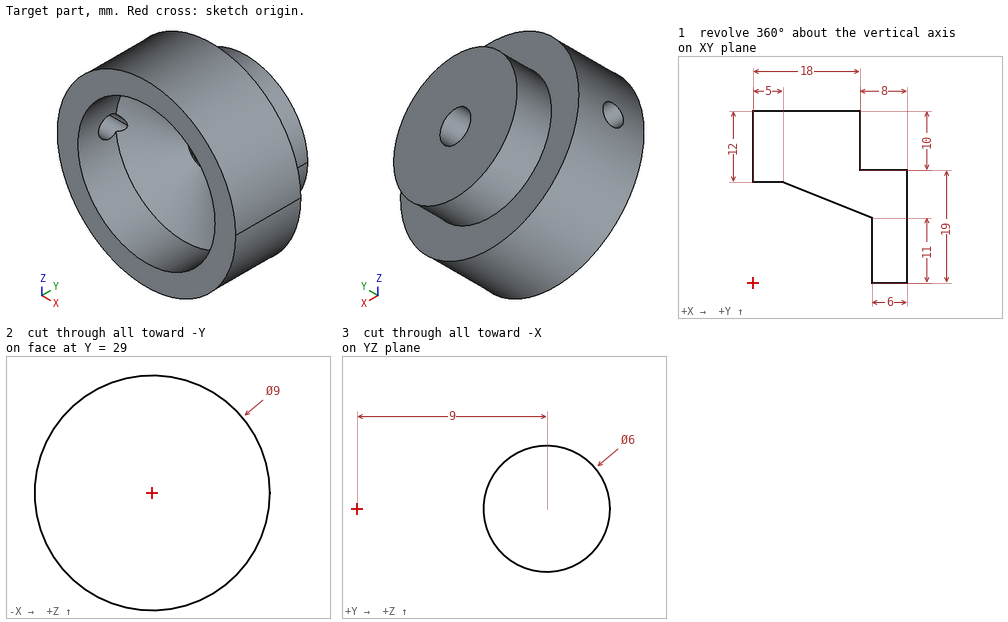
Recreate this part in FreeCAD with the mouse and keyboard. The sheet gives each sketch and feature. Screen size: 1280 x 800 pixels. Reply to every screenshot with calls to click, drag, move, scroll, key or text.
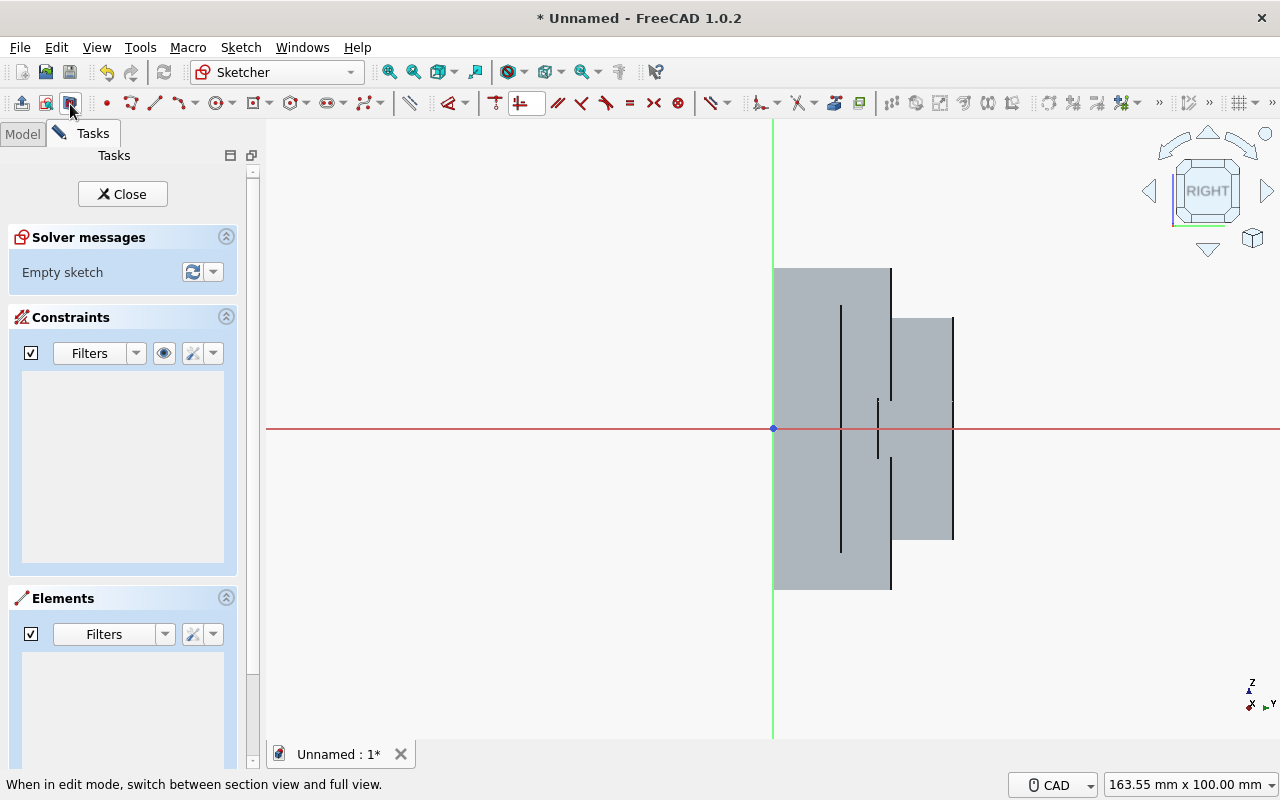
scroll(827, 429, up, 10)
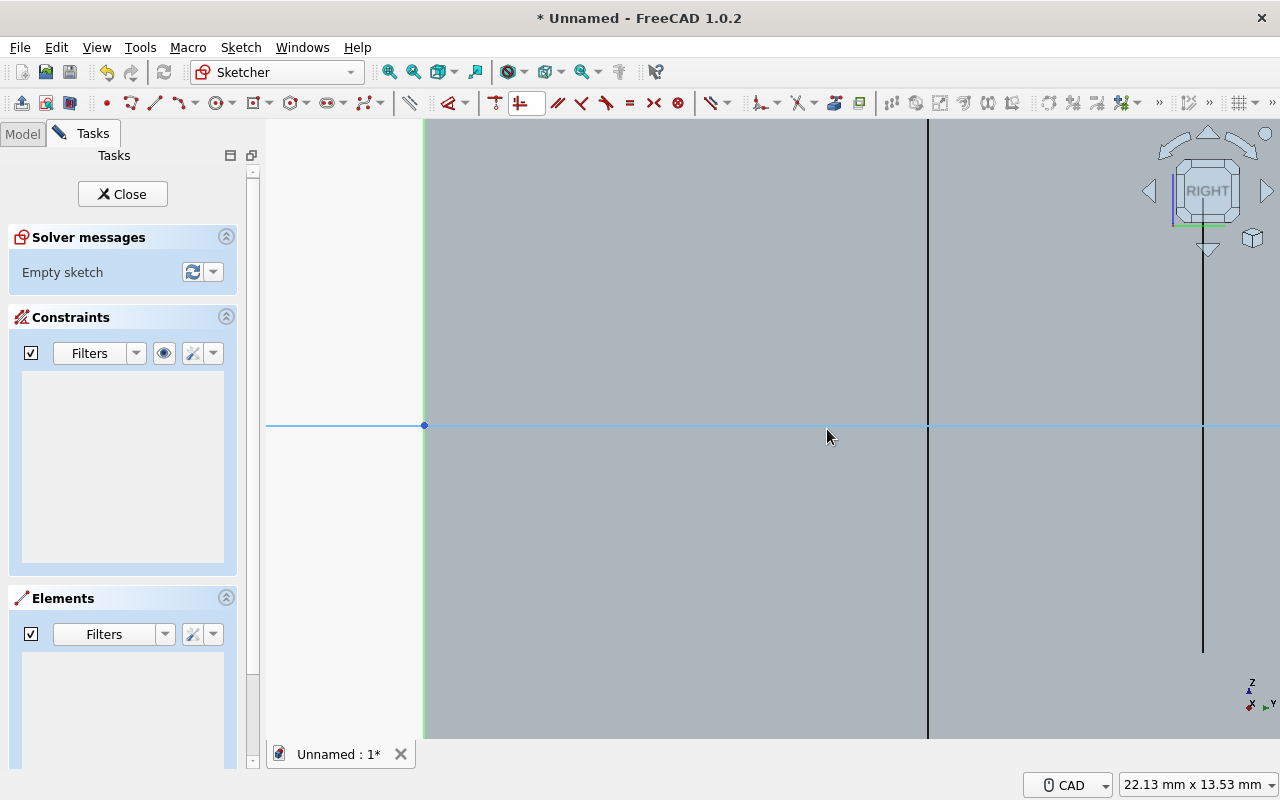
click(216, 104)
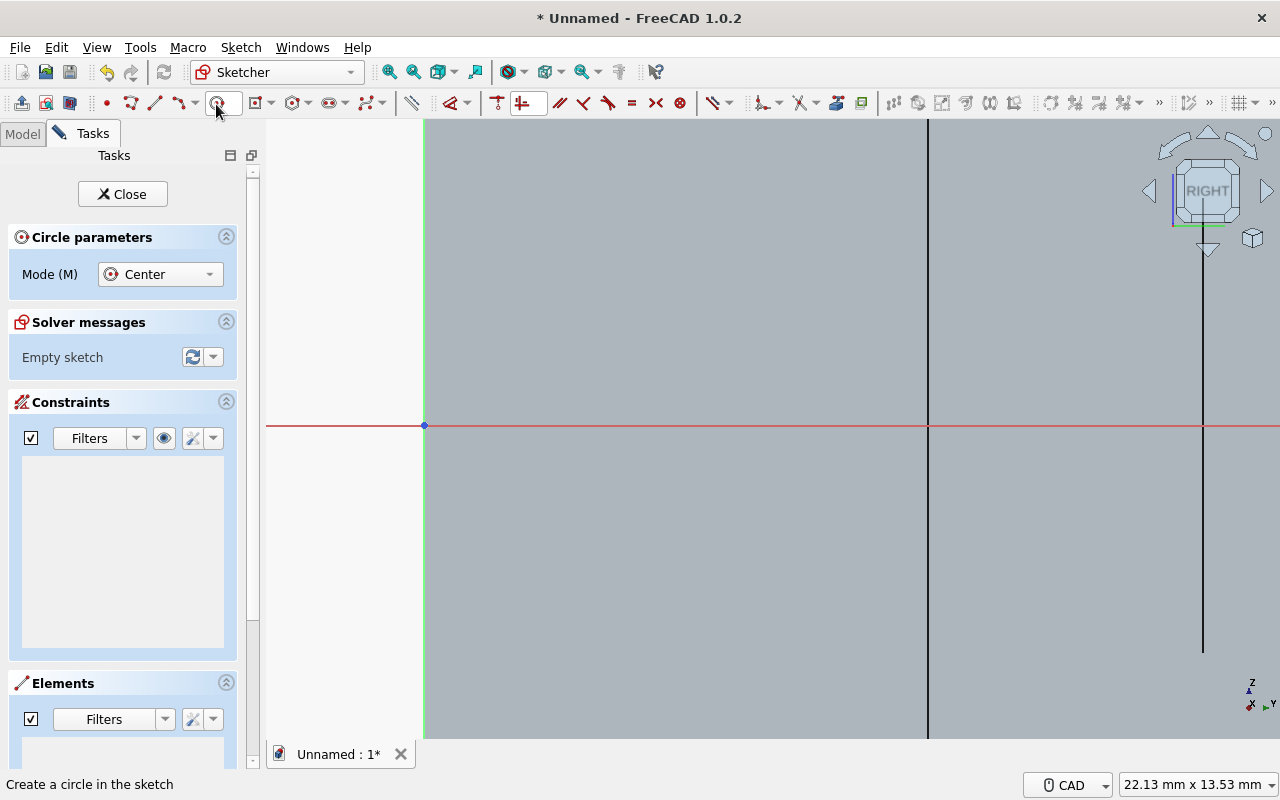
click(837, 426)
click(934, 329)
key(Escape)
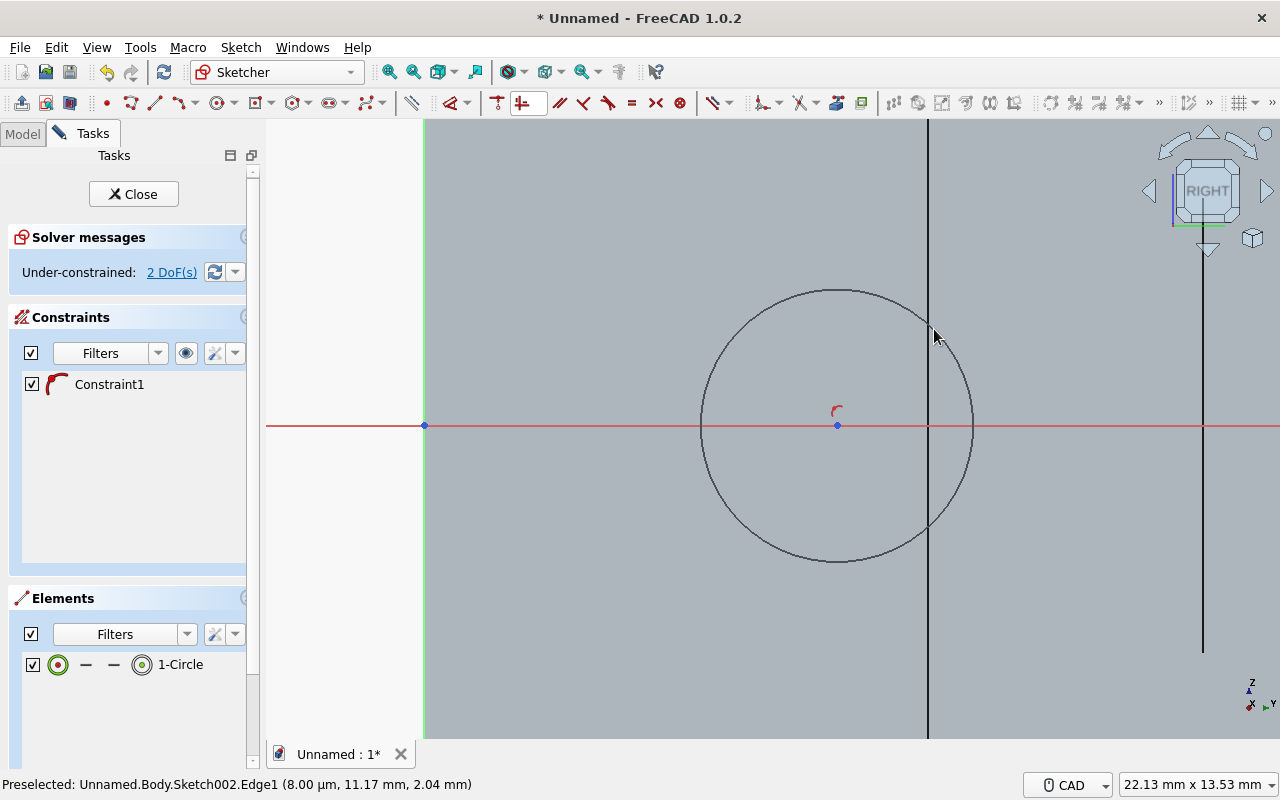
click(450, 104)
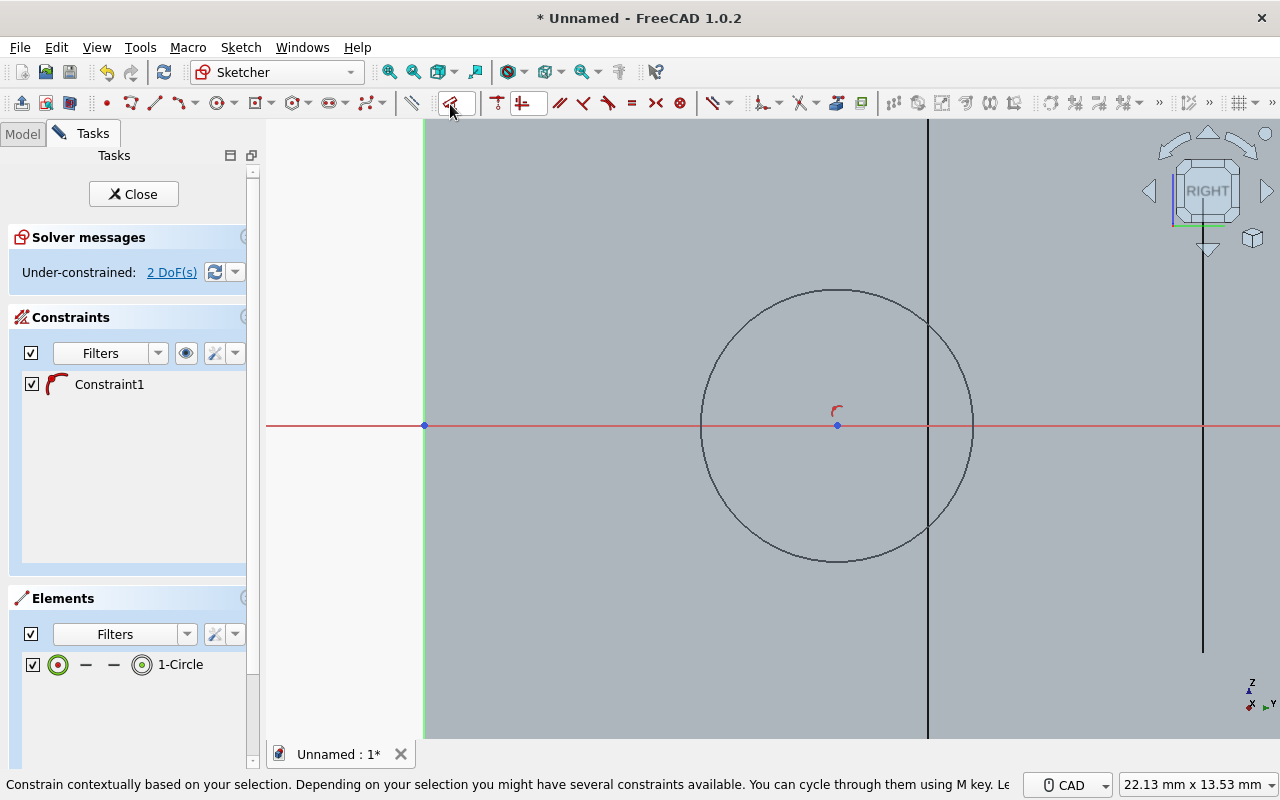
click(933, 329)
click(956, 306)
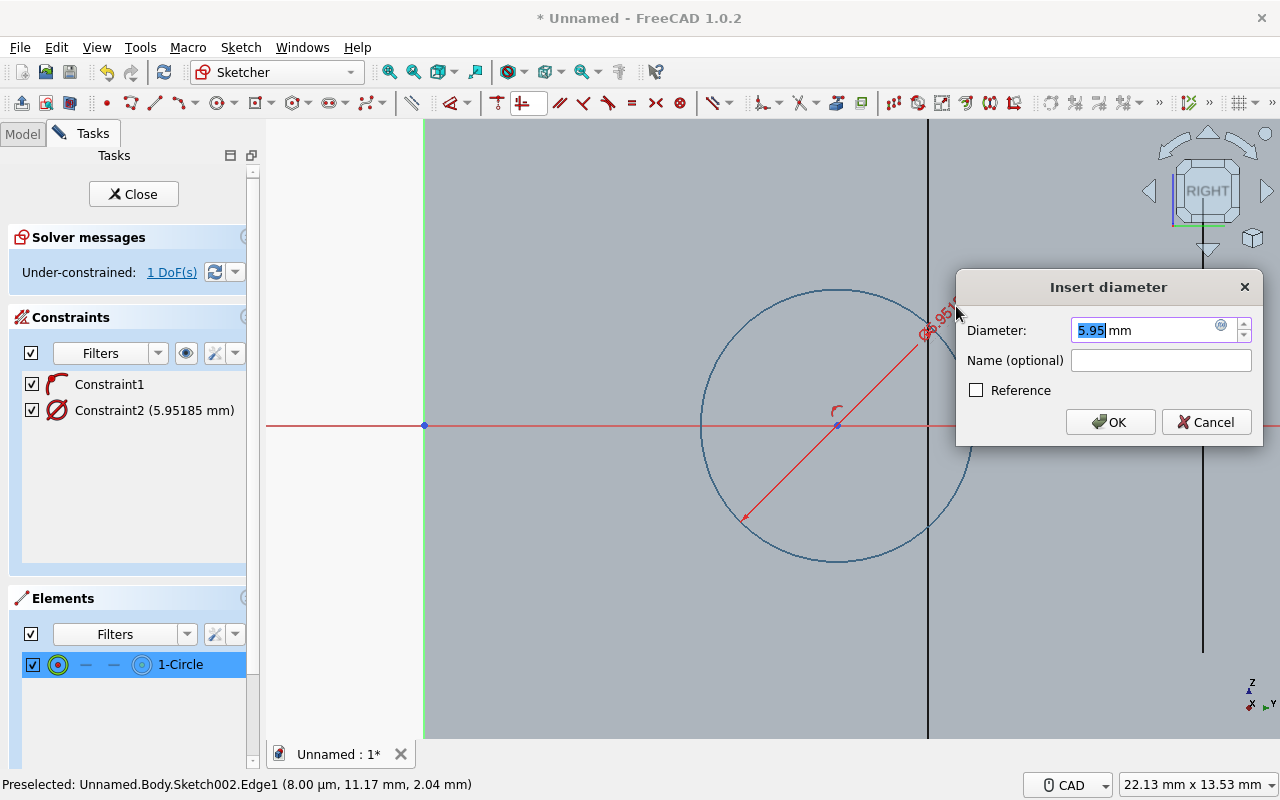
text(6)
key(Return)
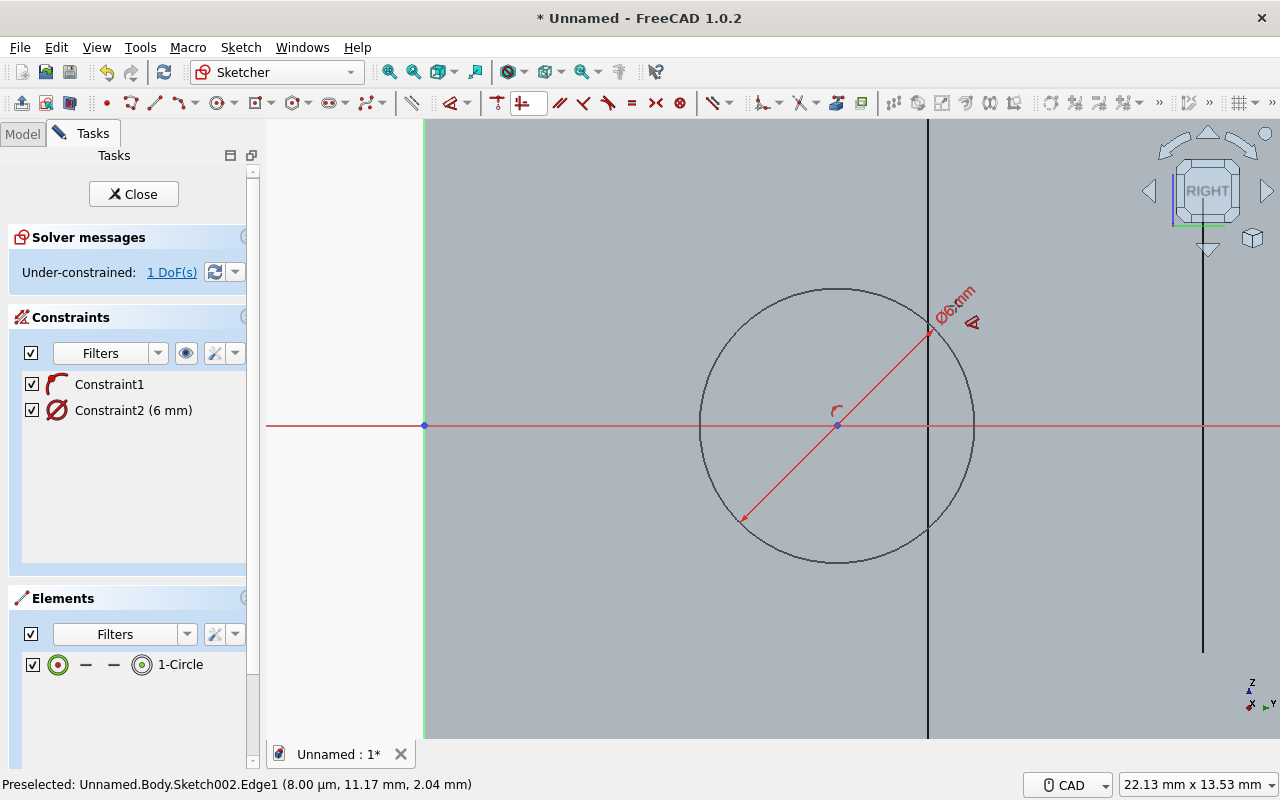
click(837, 426)
click(631, 460)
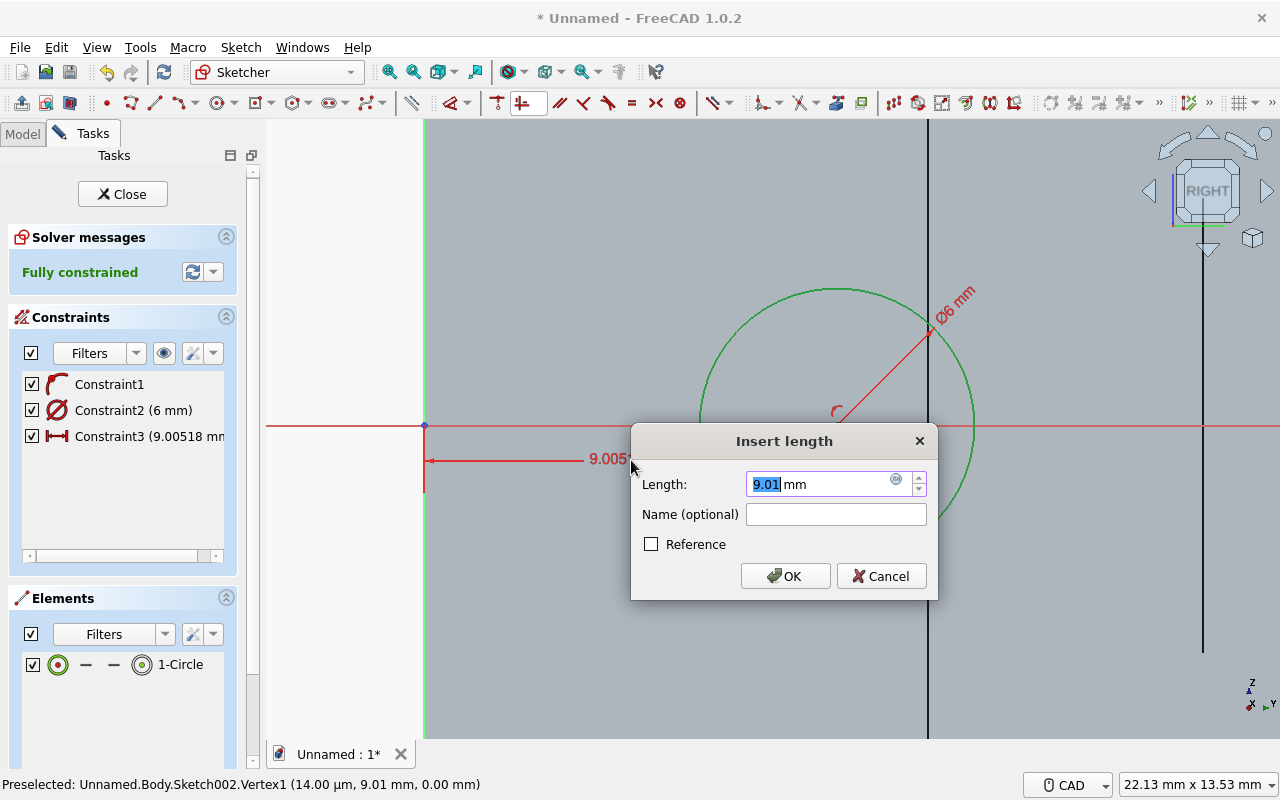
text(9)
key(Return)
key(Escape)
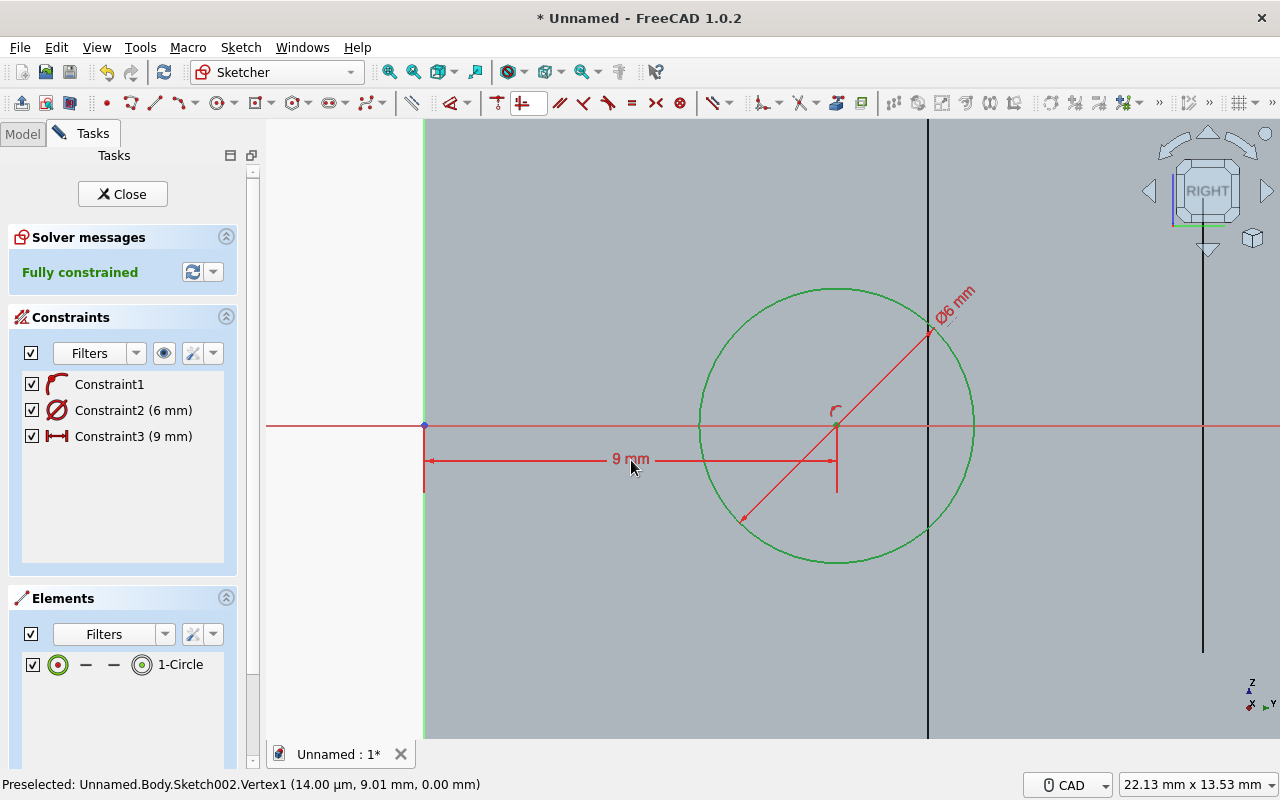
click(123, 194)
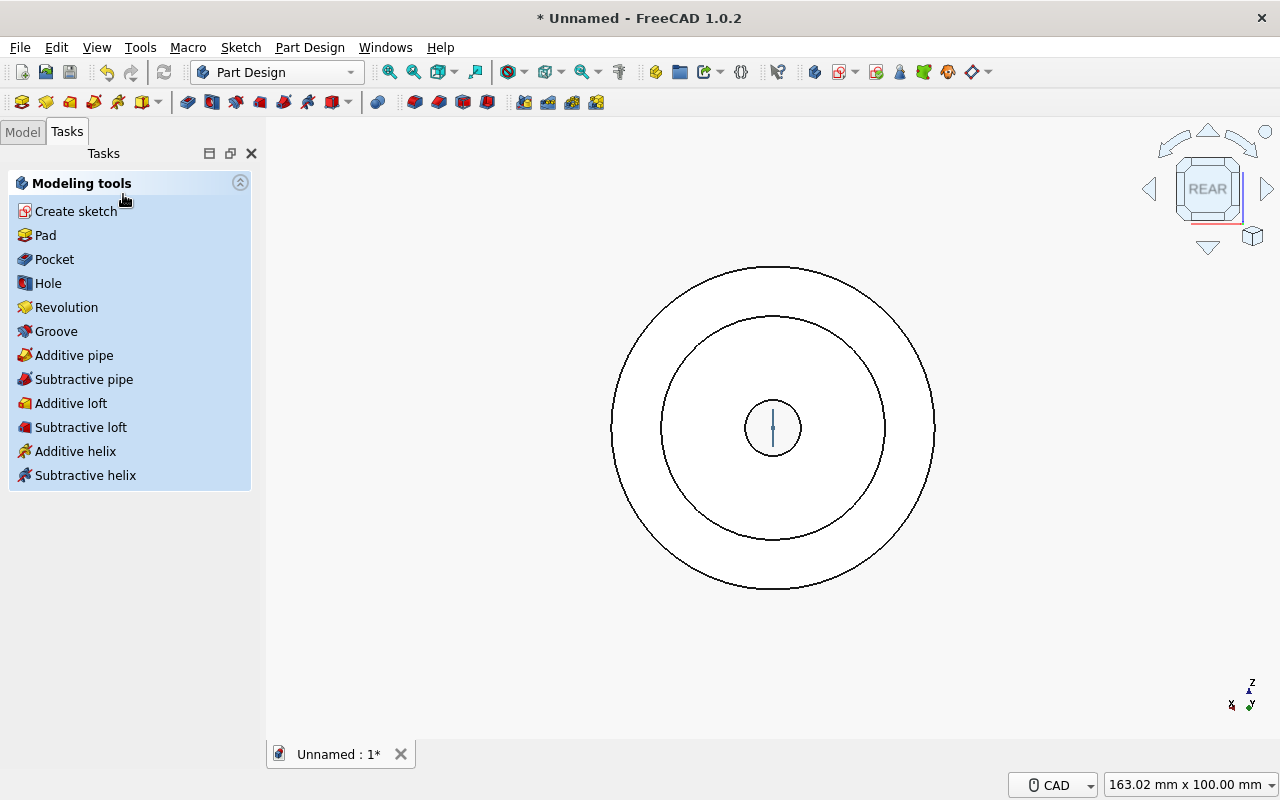
click(188, 102)